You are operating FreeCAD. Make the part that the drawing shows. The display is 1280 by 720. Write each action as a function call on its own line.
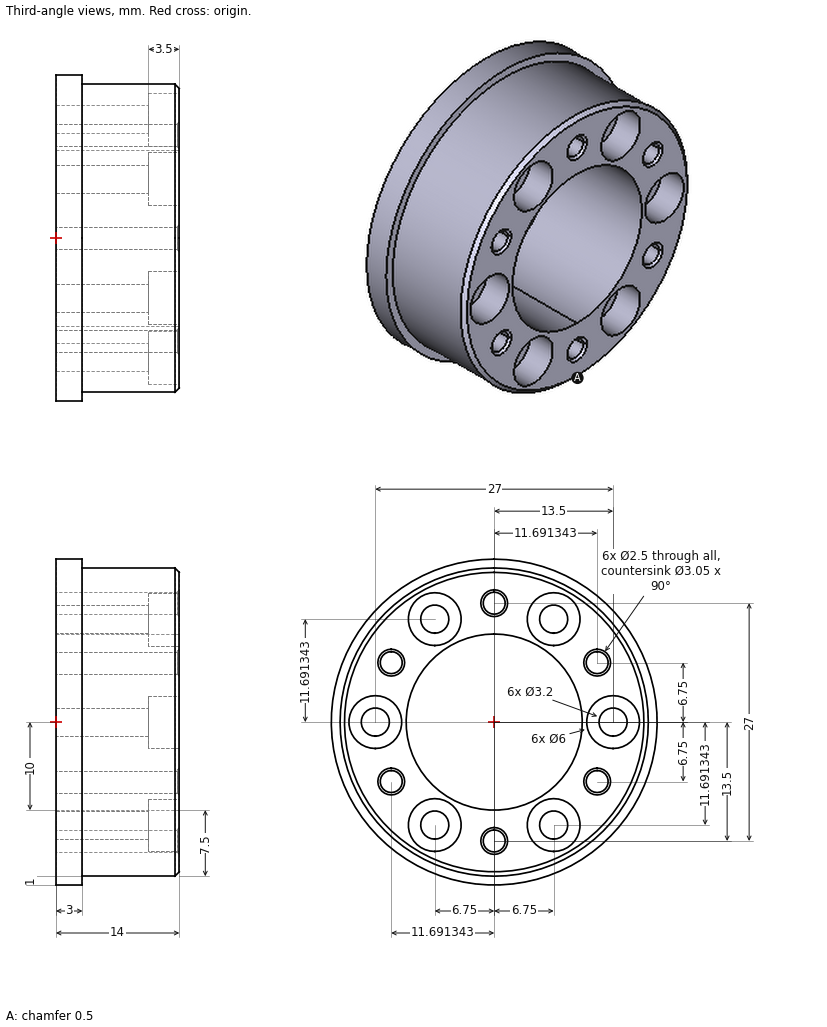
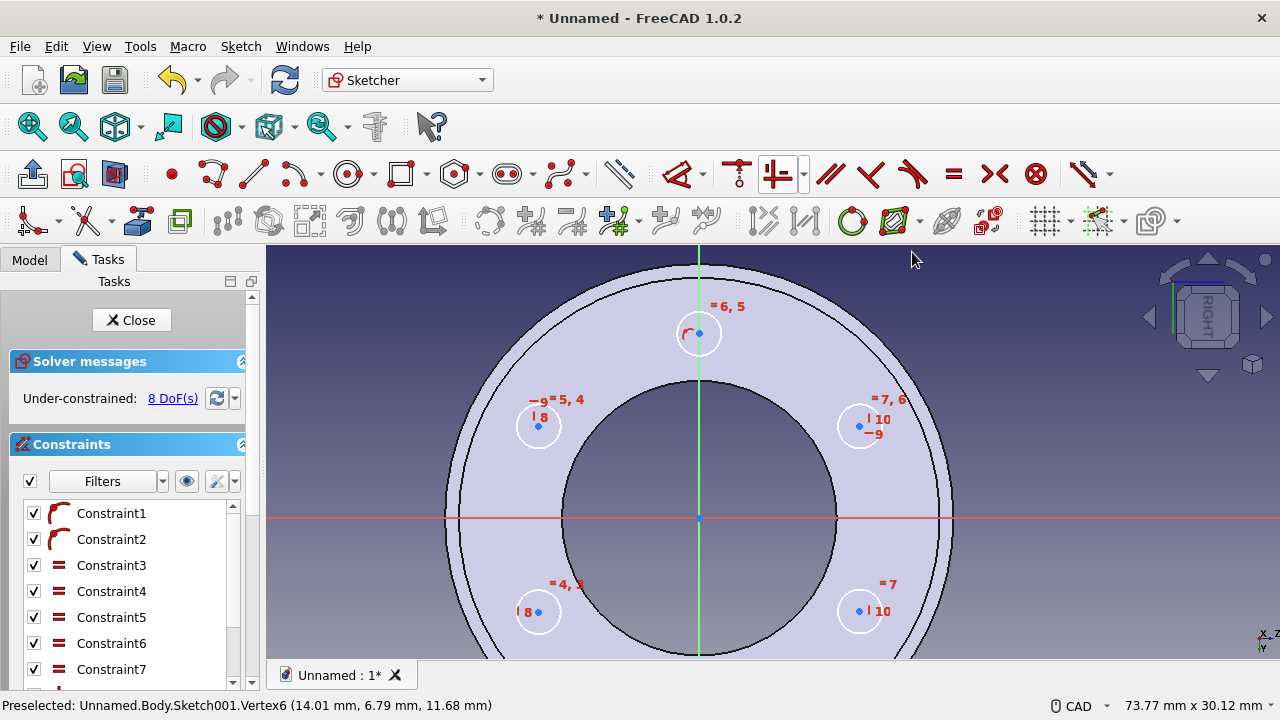
click(539, 612)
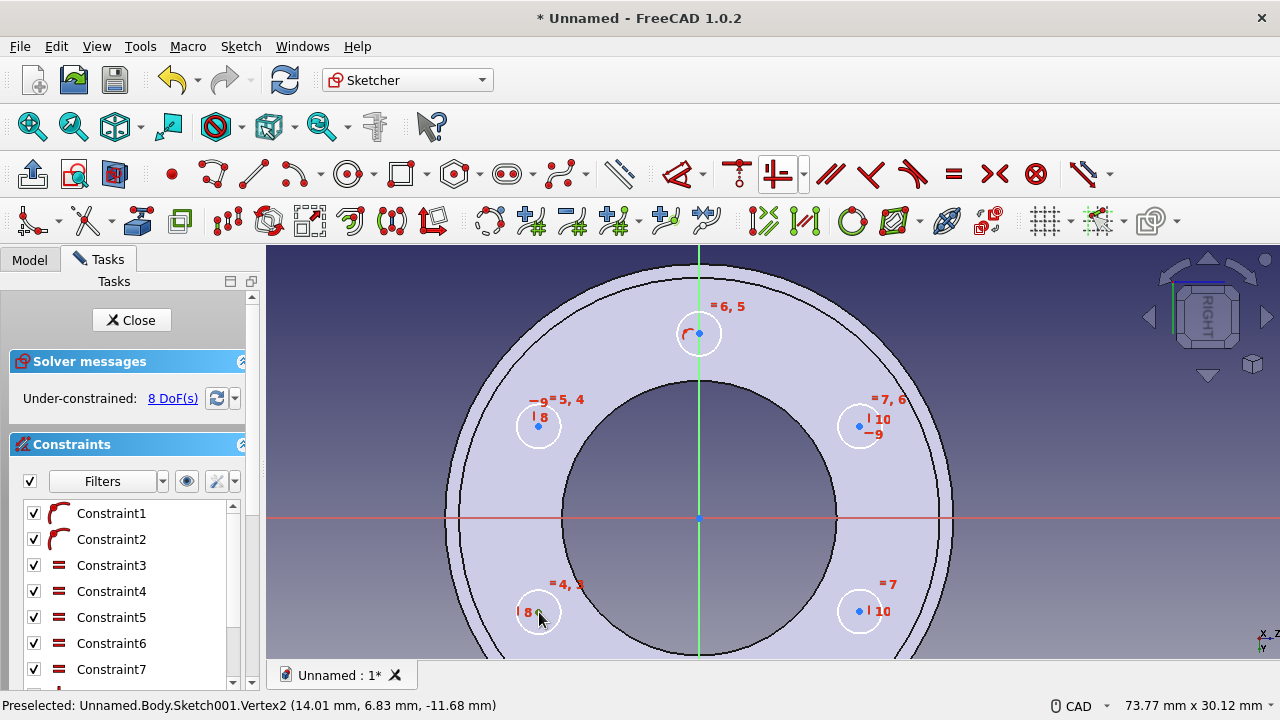
click(860, 612)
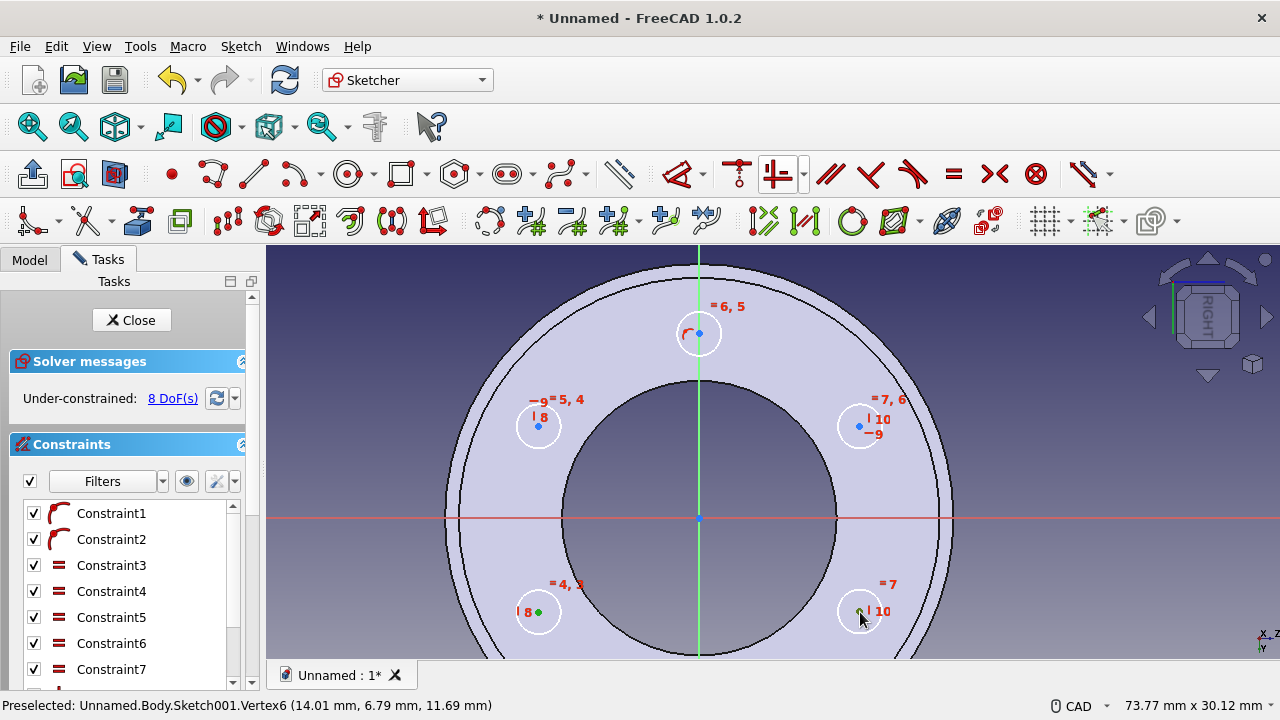
key(h)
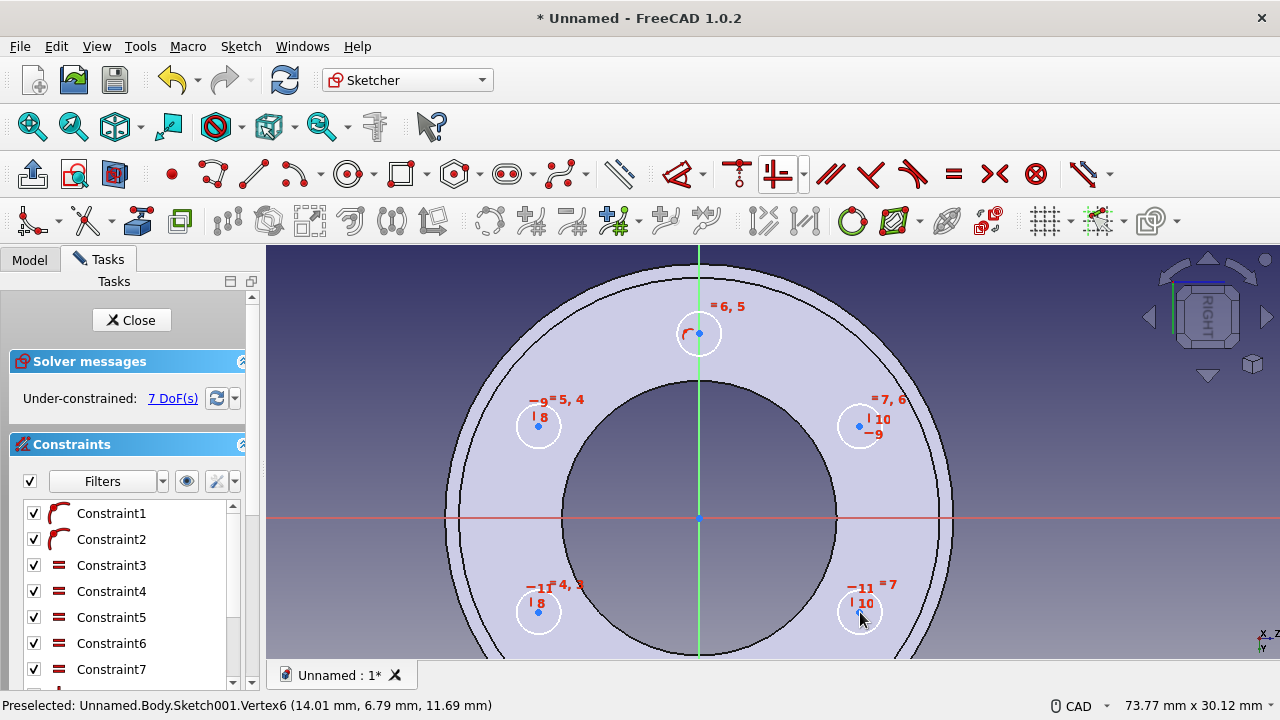
click(676, 174)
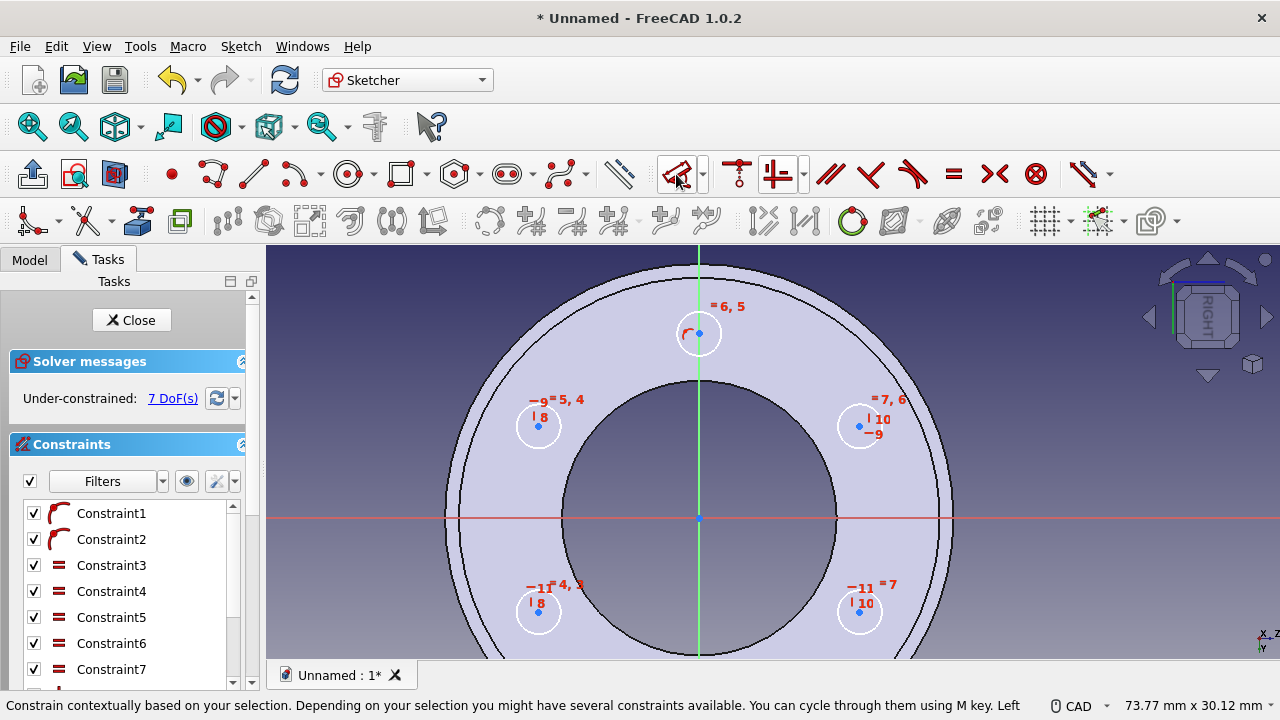
scroll(715, 317, down, 2)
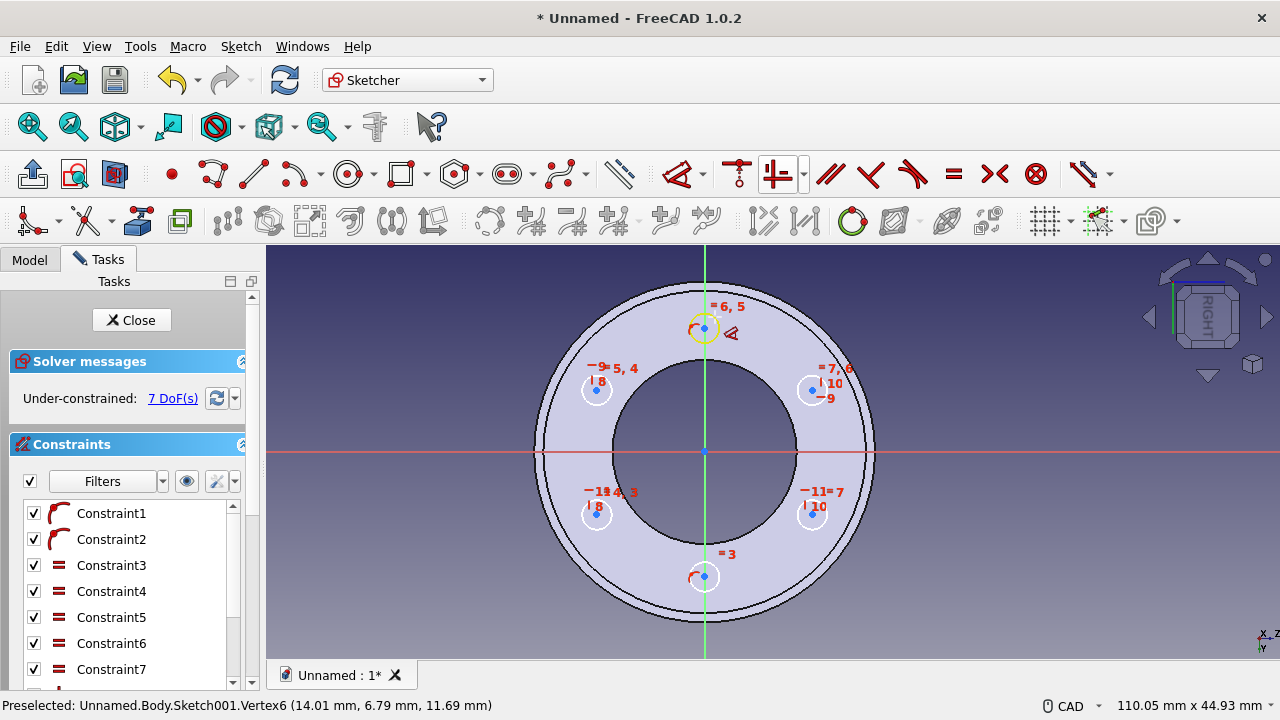
scroll(715, 566, up, 2)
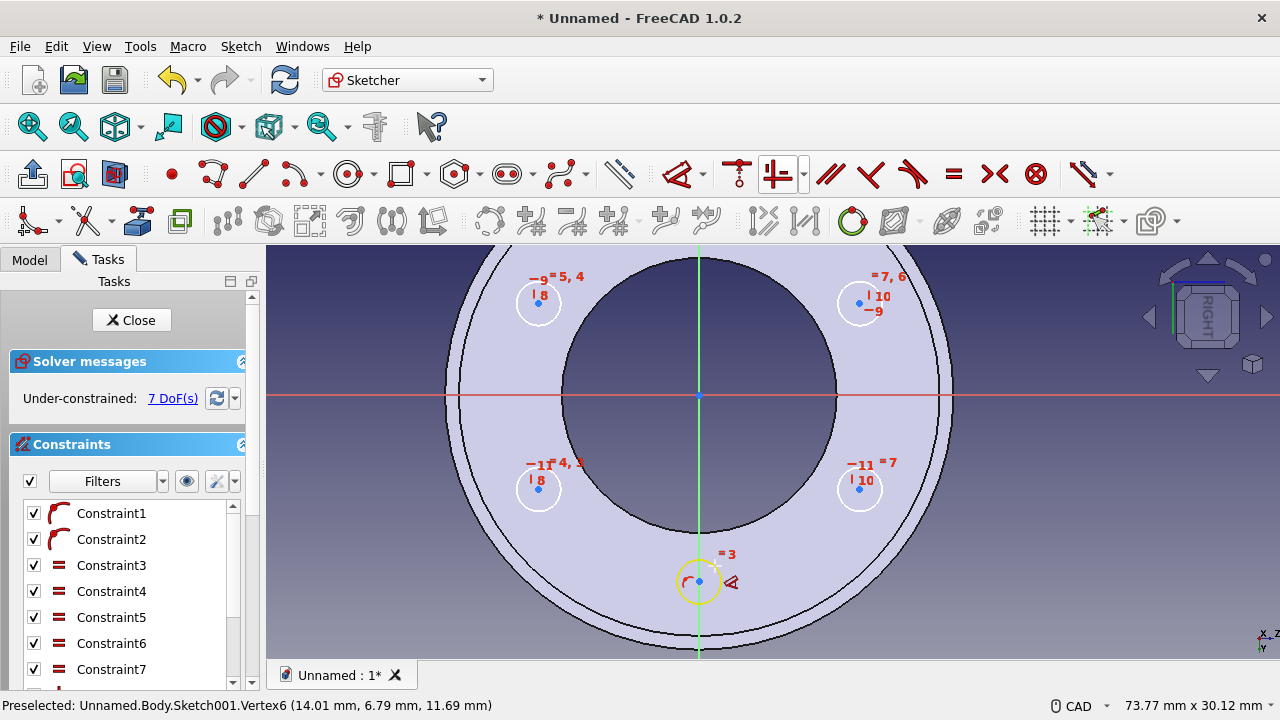
click(715, 566)
click(737, 543)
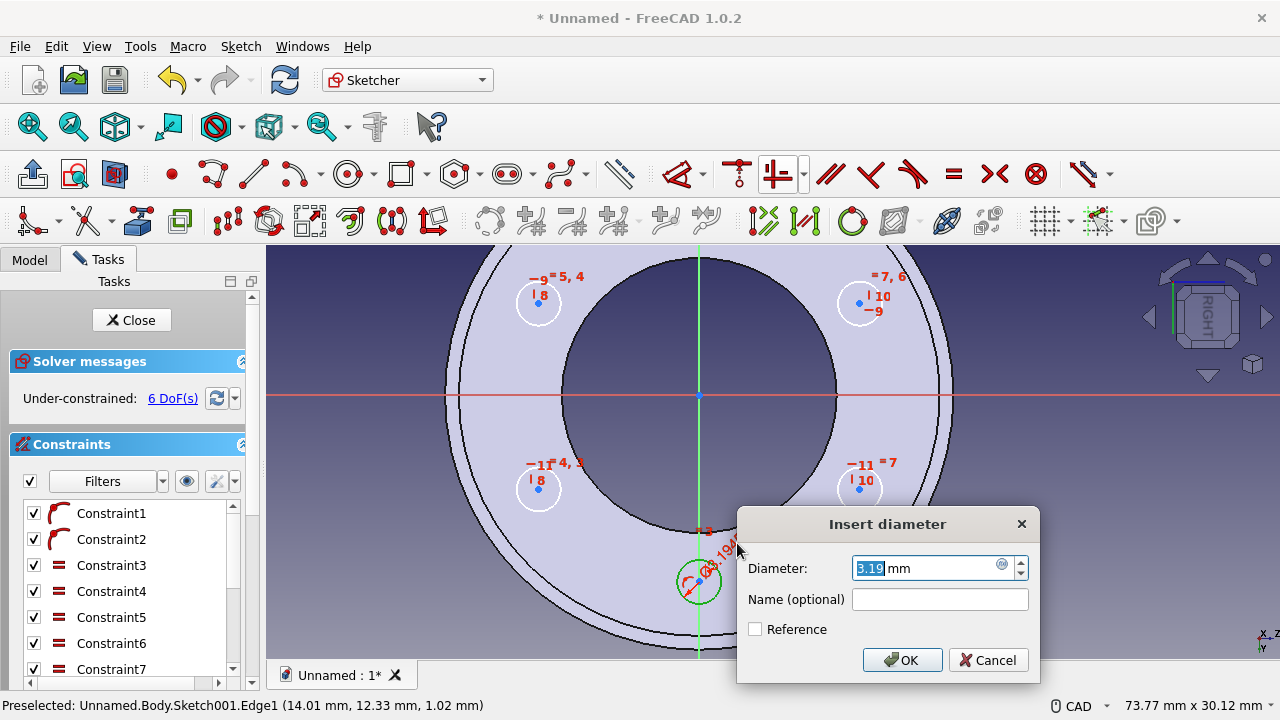
text(3.2)
key(Return)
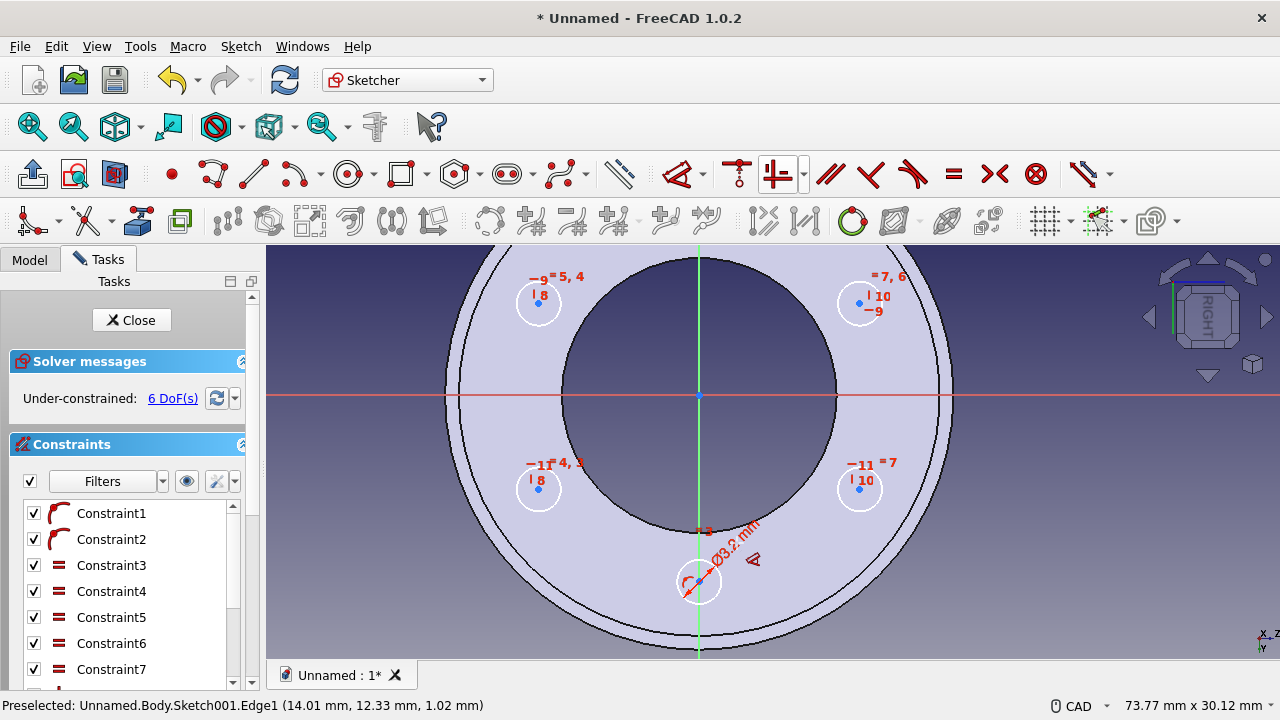
click(699, 582)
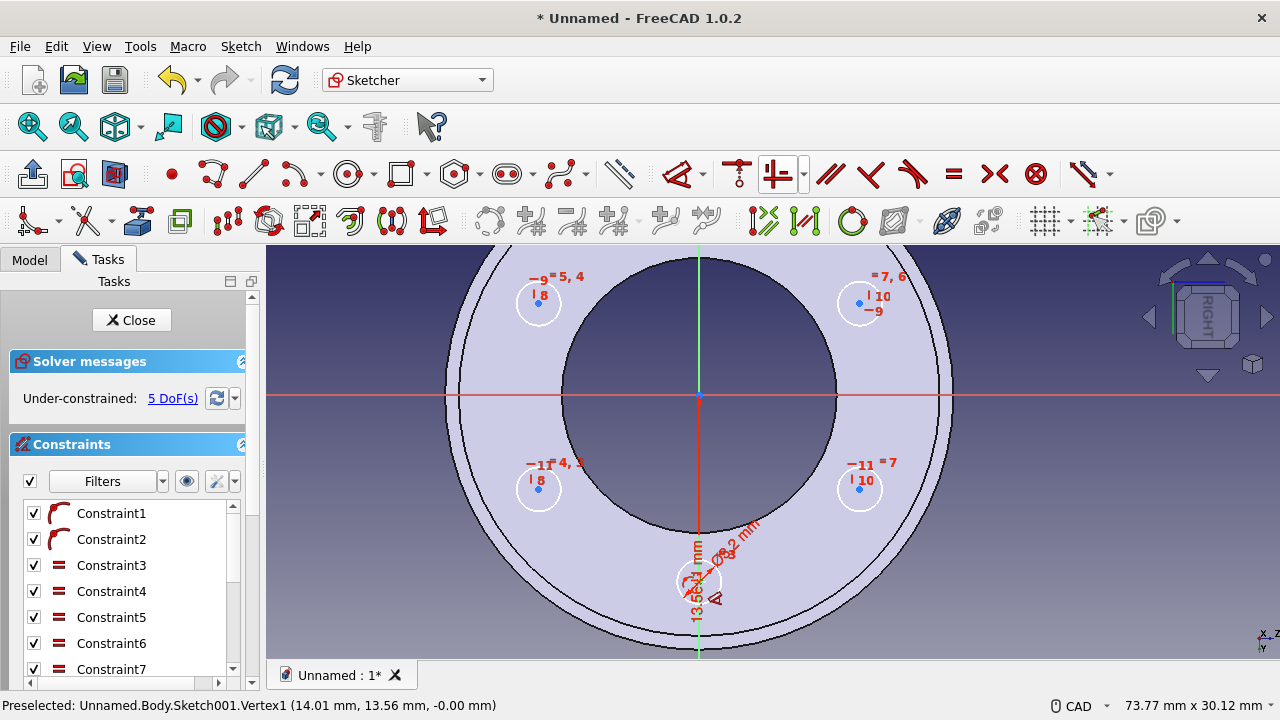
scroll(715, 567, down, 2)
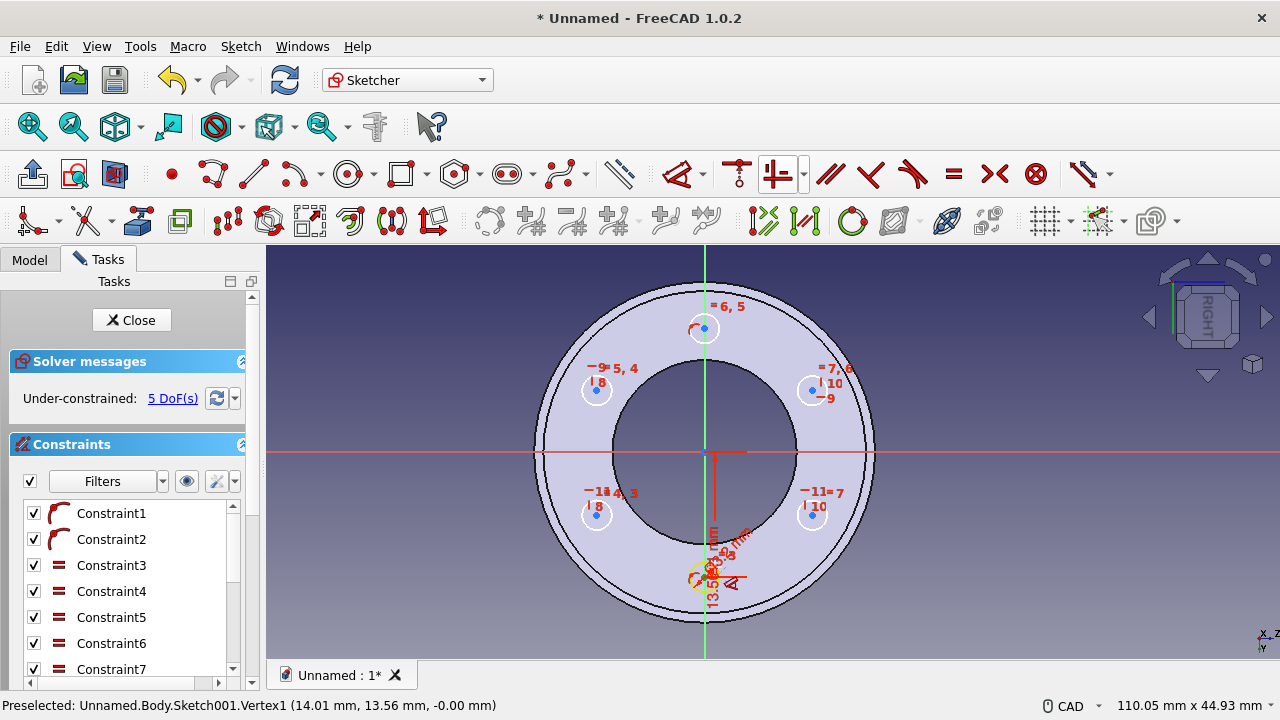
click(705, 329)
click(739, 396)